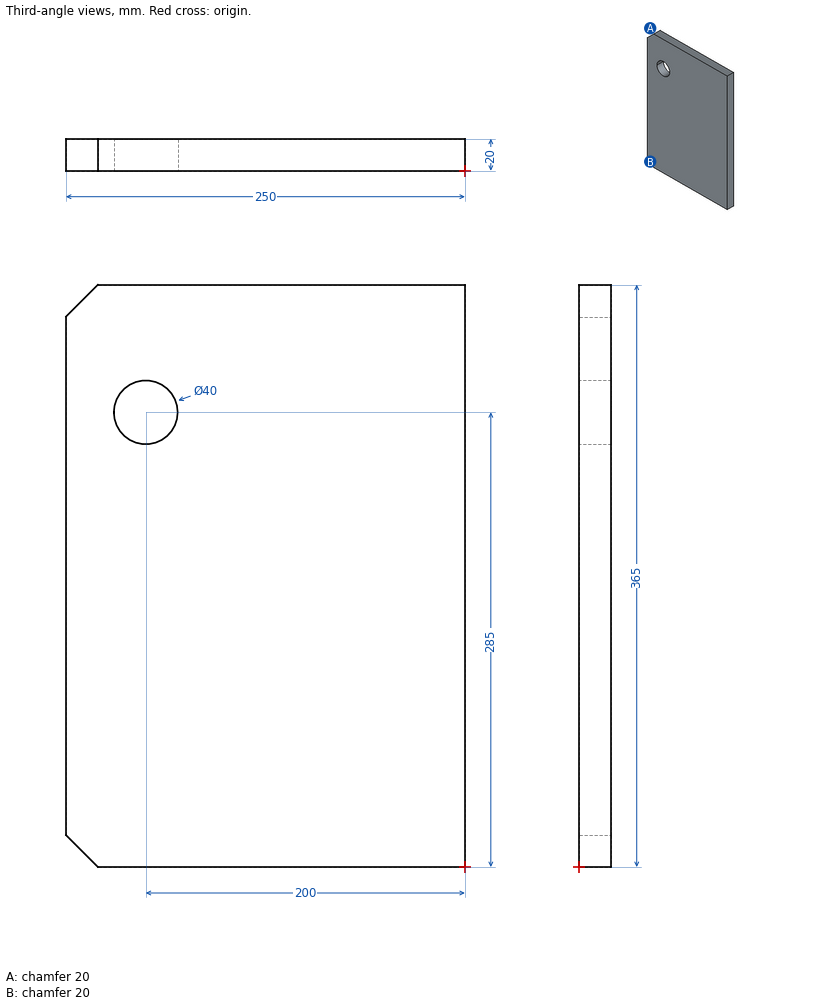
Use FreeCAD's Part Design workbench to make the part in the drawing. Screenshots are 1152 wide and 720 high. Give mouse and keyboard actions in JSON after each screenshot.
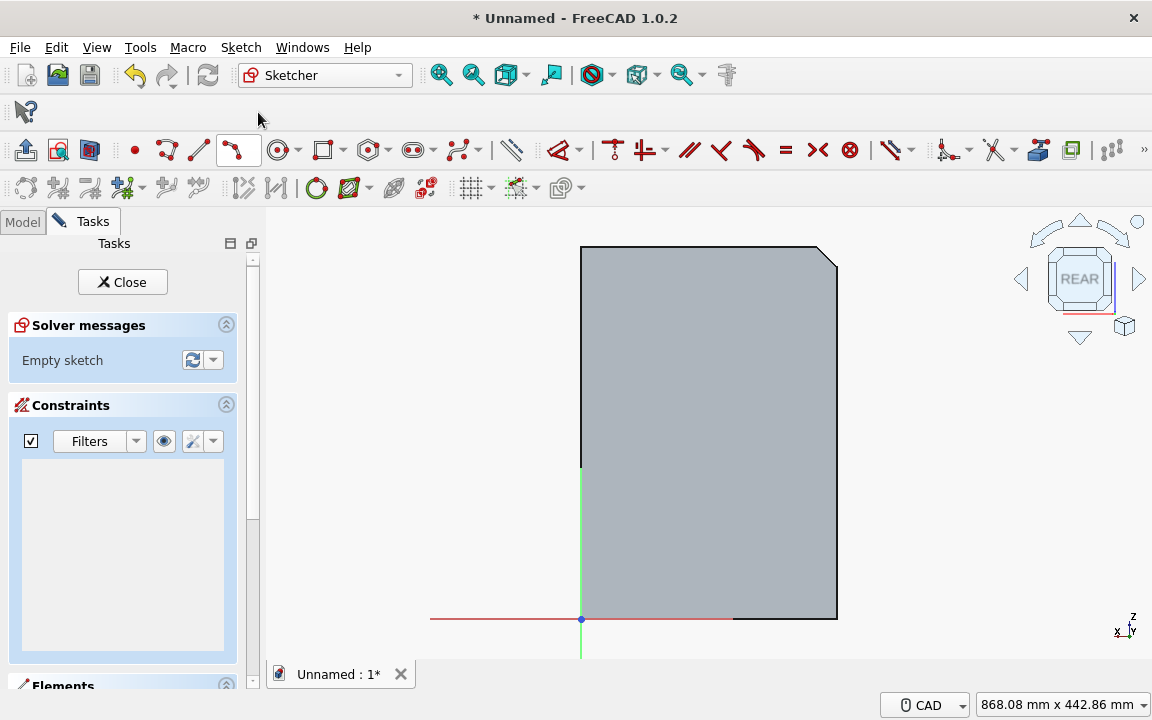
{"action": "scroll", "coordinate": [808, 312], "scroll_direction": "up", "scroll_amount": 10}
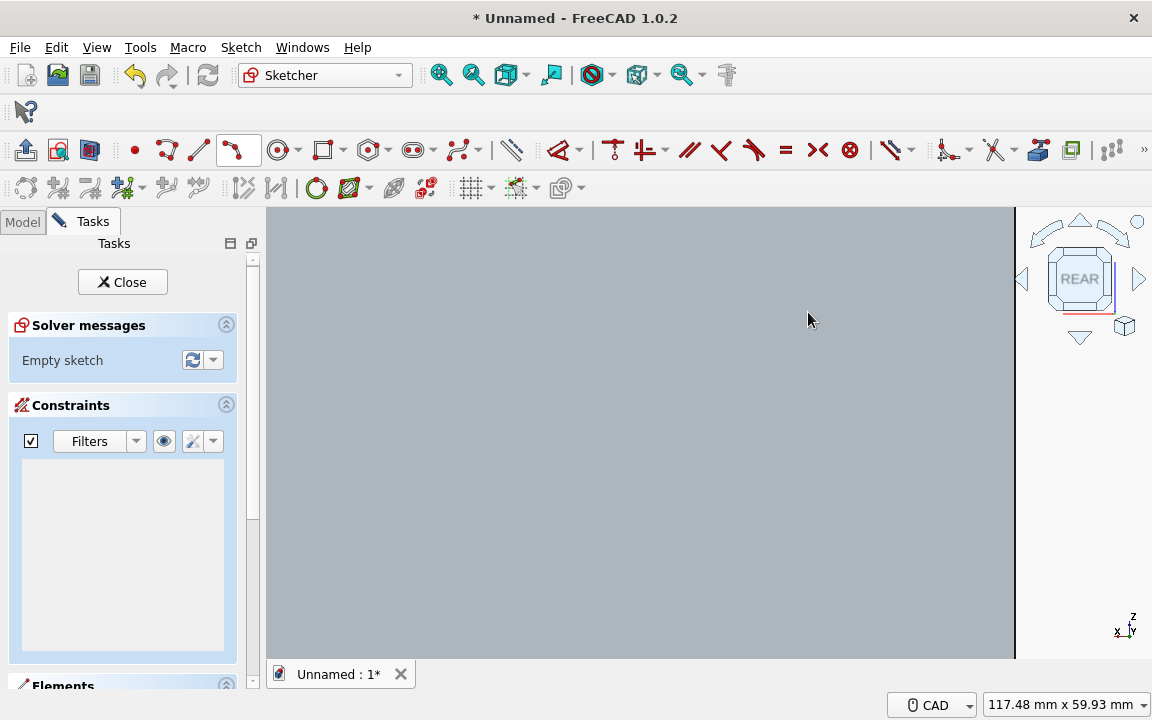
{"action": "key", "text": "g c"}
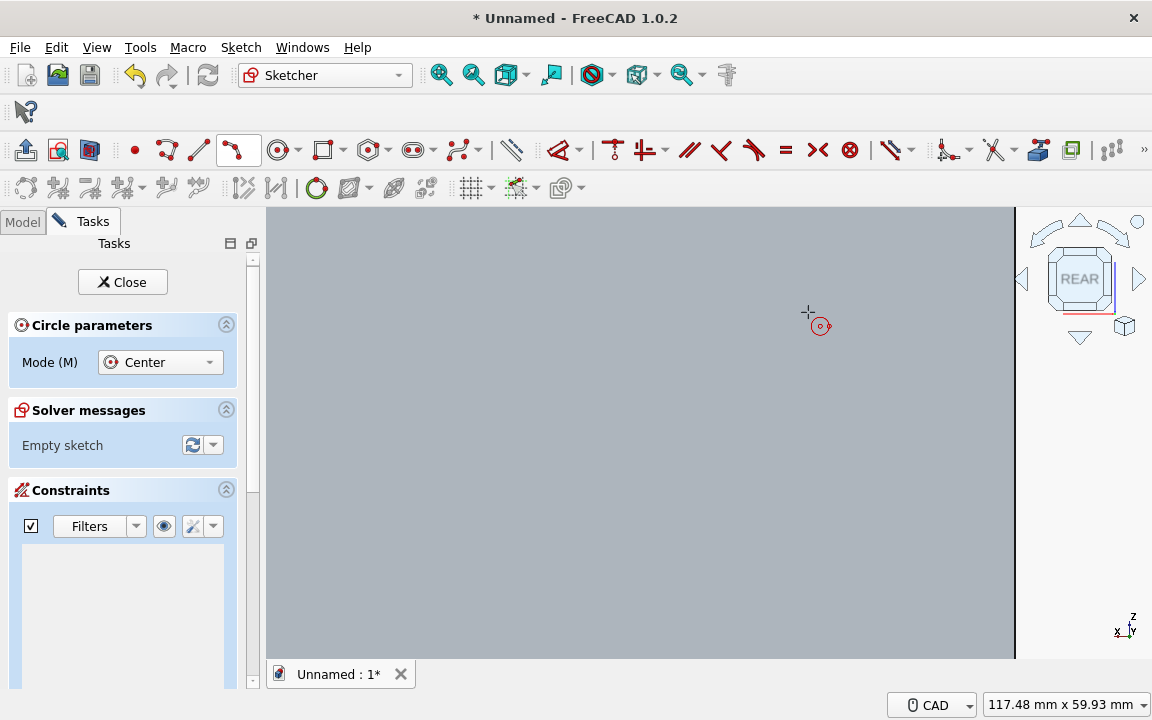
{"action": "left_click", "coordinate": [638, 432]}
{"action": "mouse_move", "coordinate": [745, 325]}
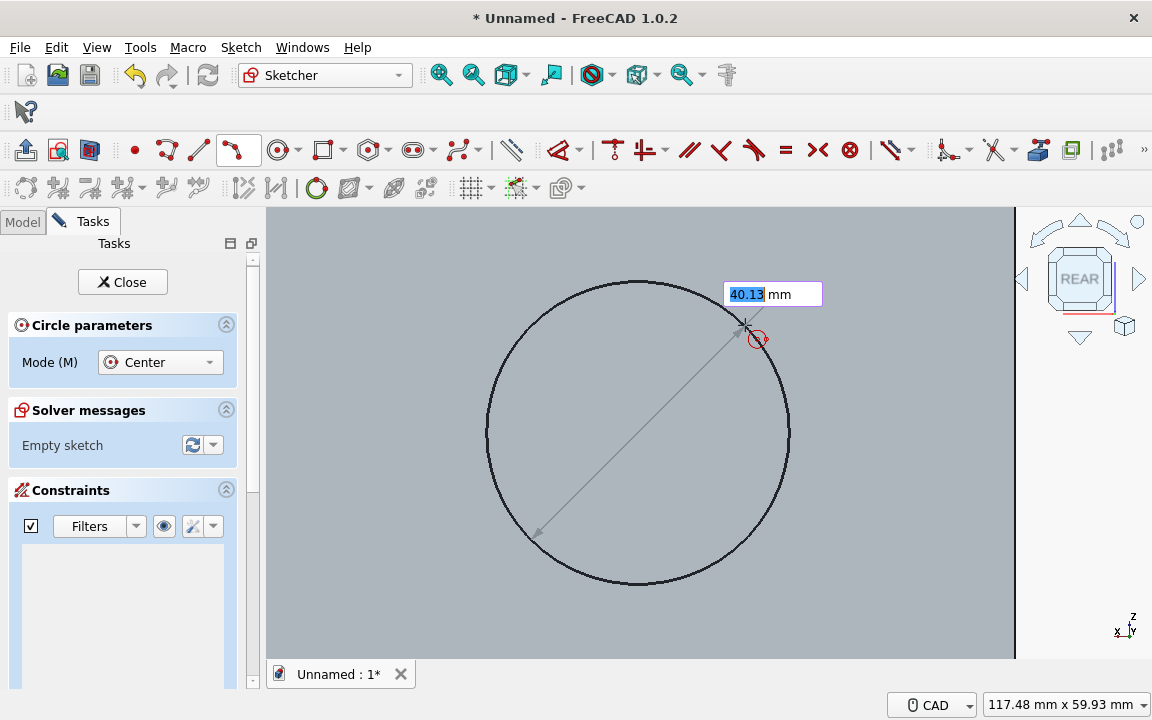
{"action": "type", "text": "40"}
{"action": "key", "text": "Return"}
{"action": "key", "text": "Escape"}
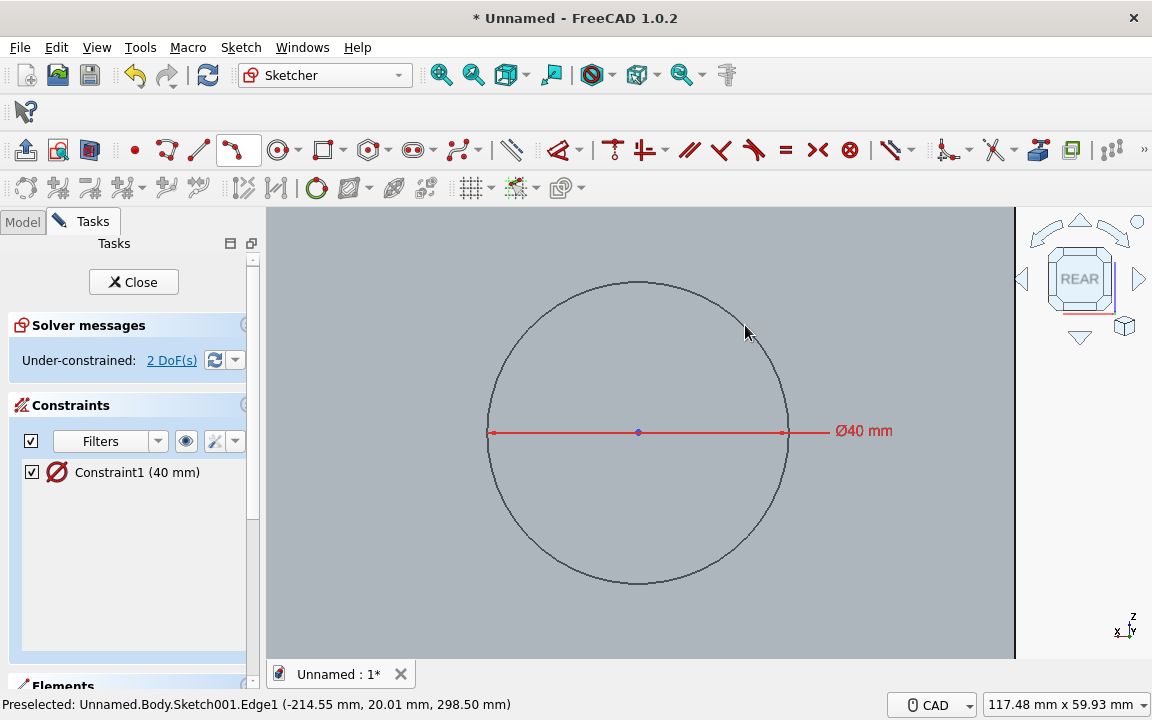
{"action": "key", "text": "d"}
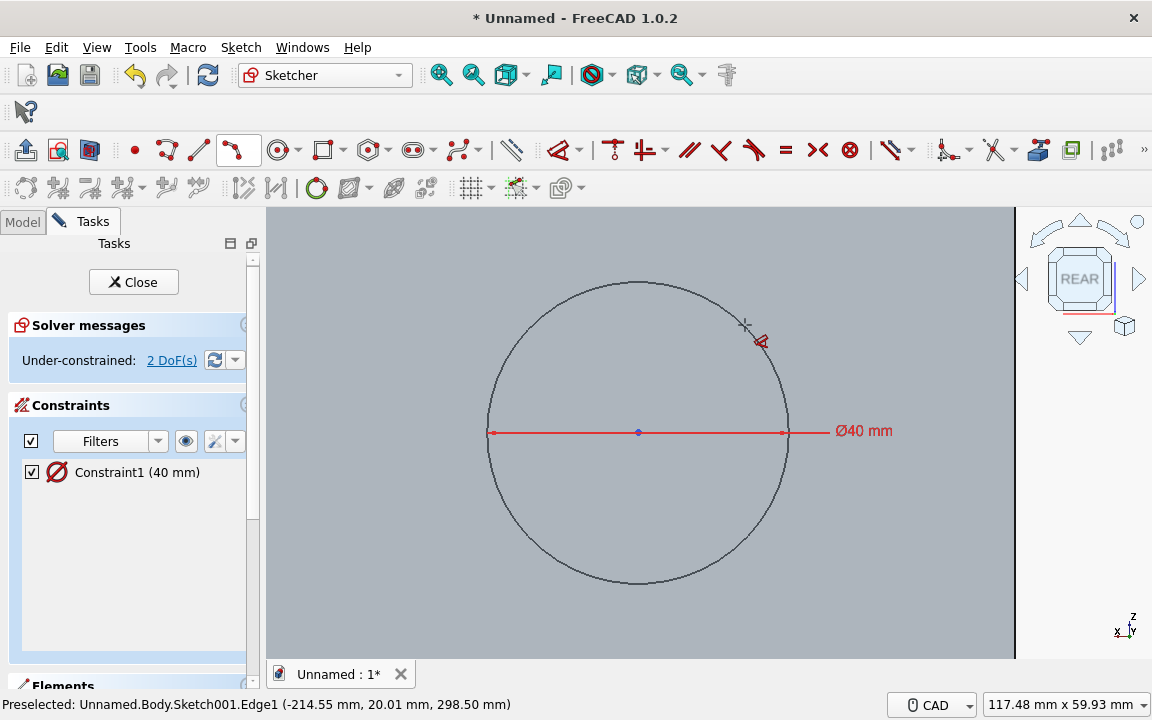
{"action": "left_click", "coordinate": [638, 433]}
{"action": "left_click", "coordinate": [466, 399]}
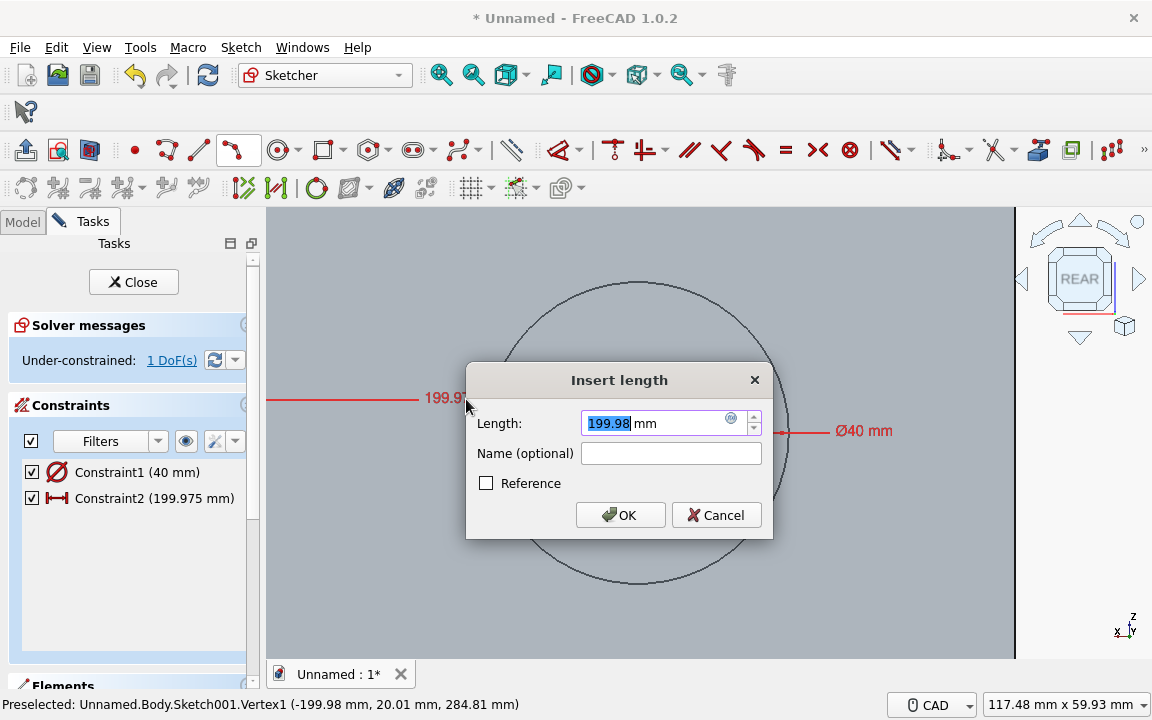
{"action": "type", "text": "200"}
{"action": "key", "text": "Return"}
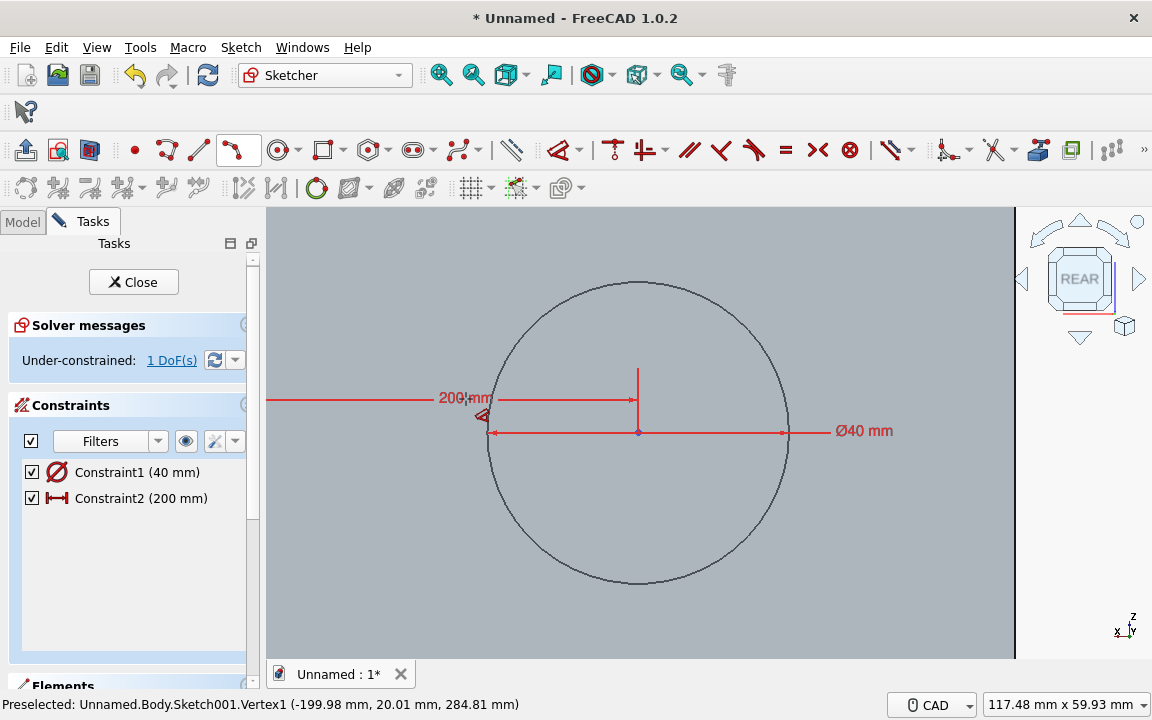
{"action": "left_click", "coordinate": [638, 433]}
{"action": "left_click", "coordinate": [672, 532]}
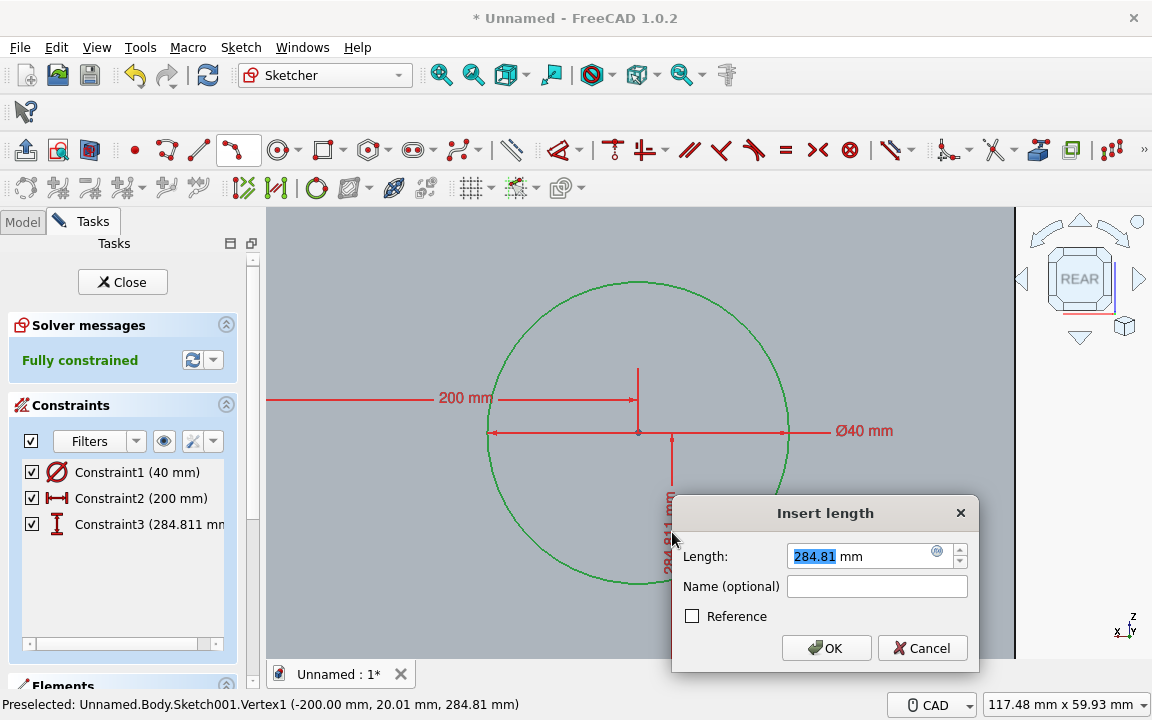
{"action": "type", "text": "285"}
{"action": "key", "text": "Return"}
{"action": "key", "text": "Escape"}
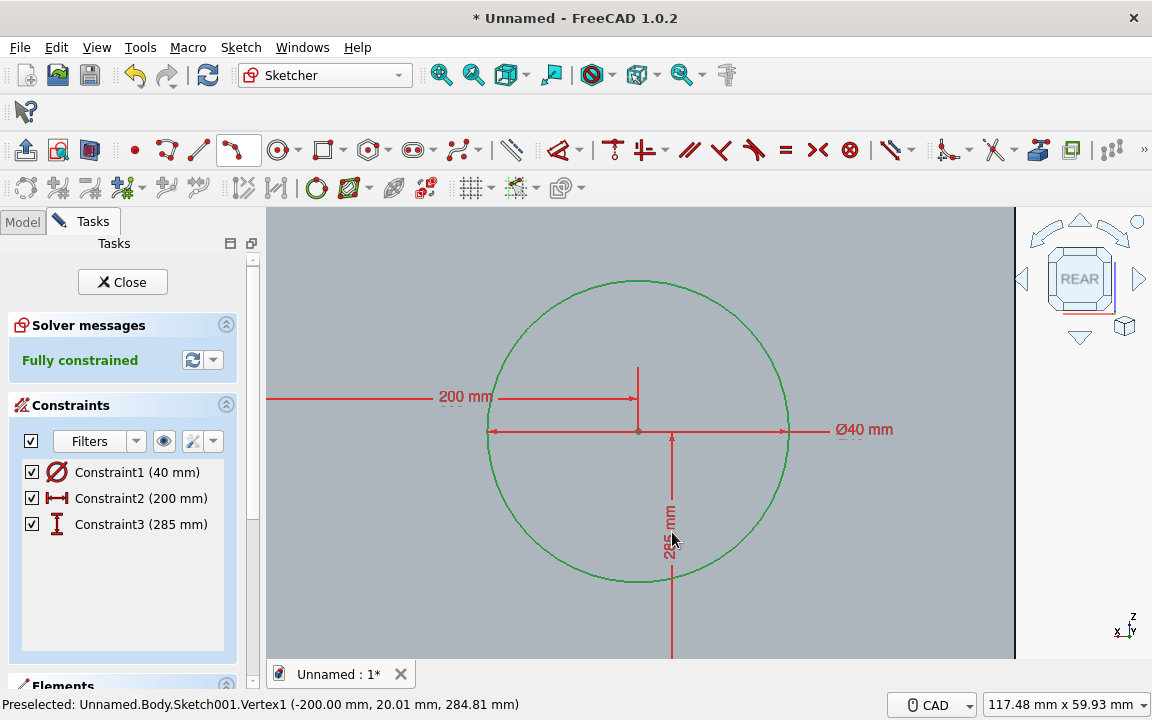
{"action": "left_click", "coordinate": [123, 282]}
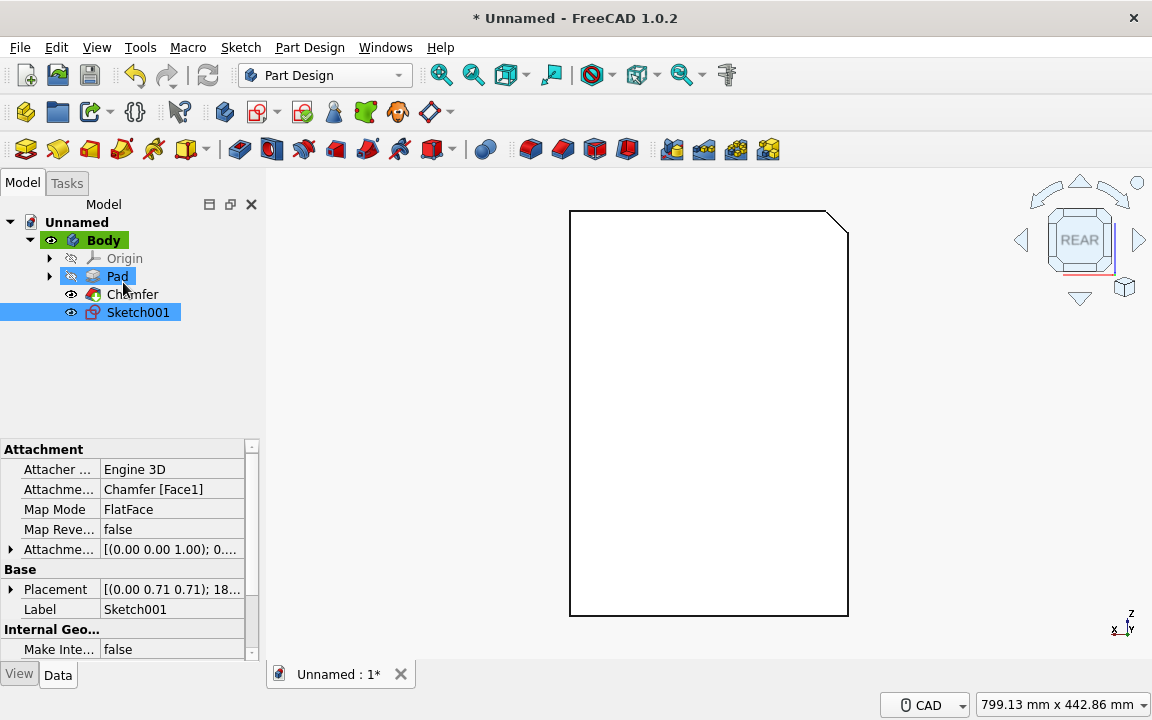
{"action": "left_click", "coordinate": [240, 150]}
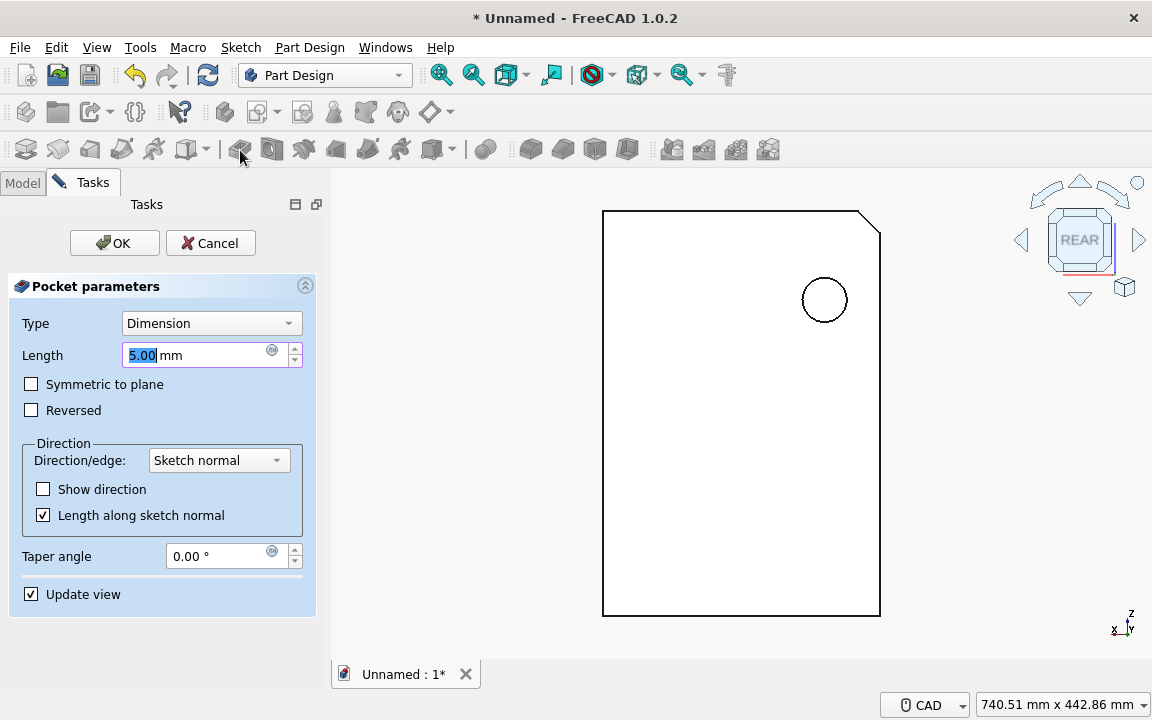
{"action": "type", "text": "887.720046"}
{"action": "key", "text": "Tab"}